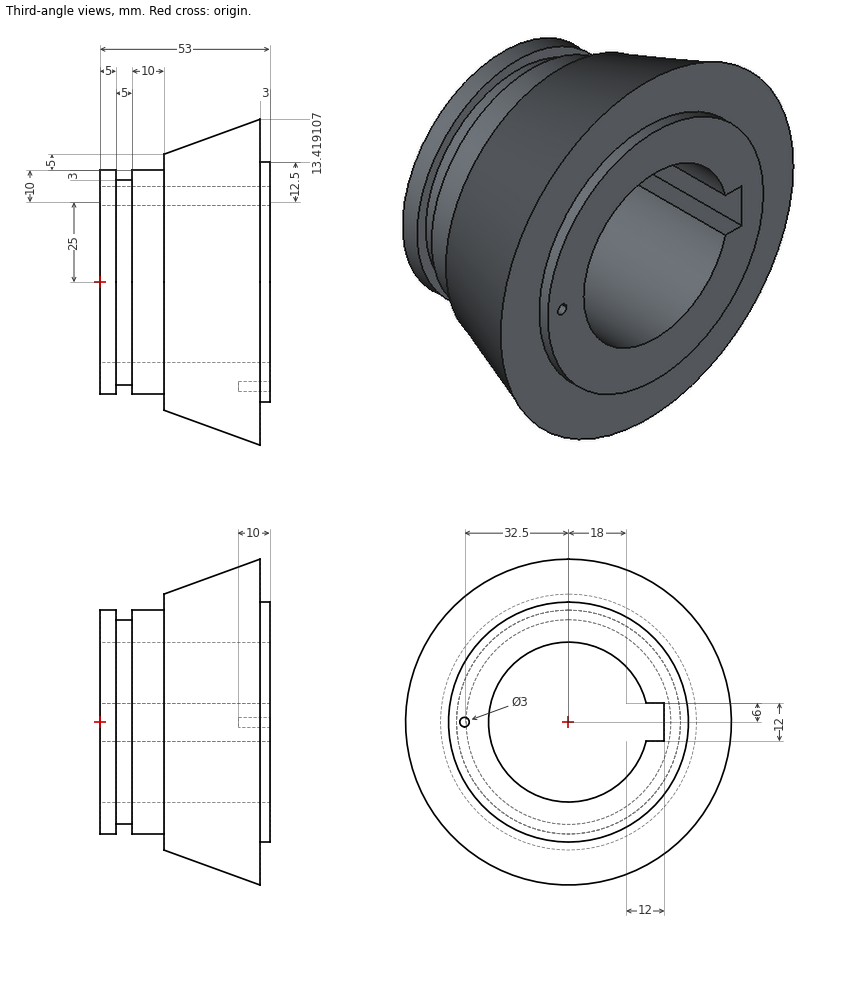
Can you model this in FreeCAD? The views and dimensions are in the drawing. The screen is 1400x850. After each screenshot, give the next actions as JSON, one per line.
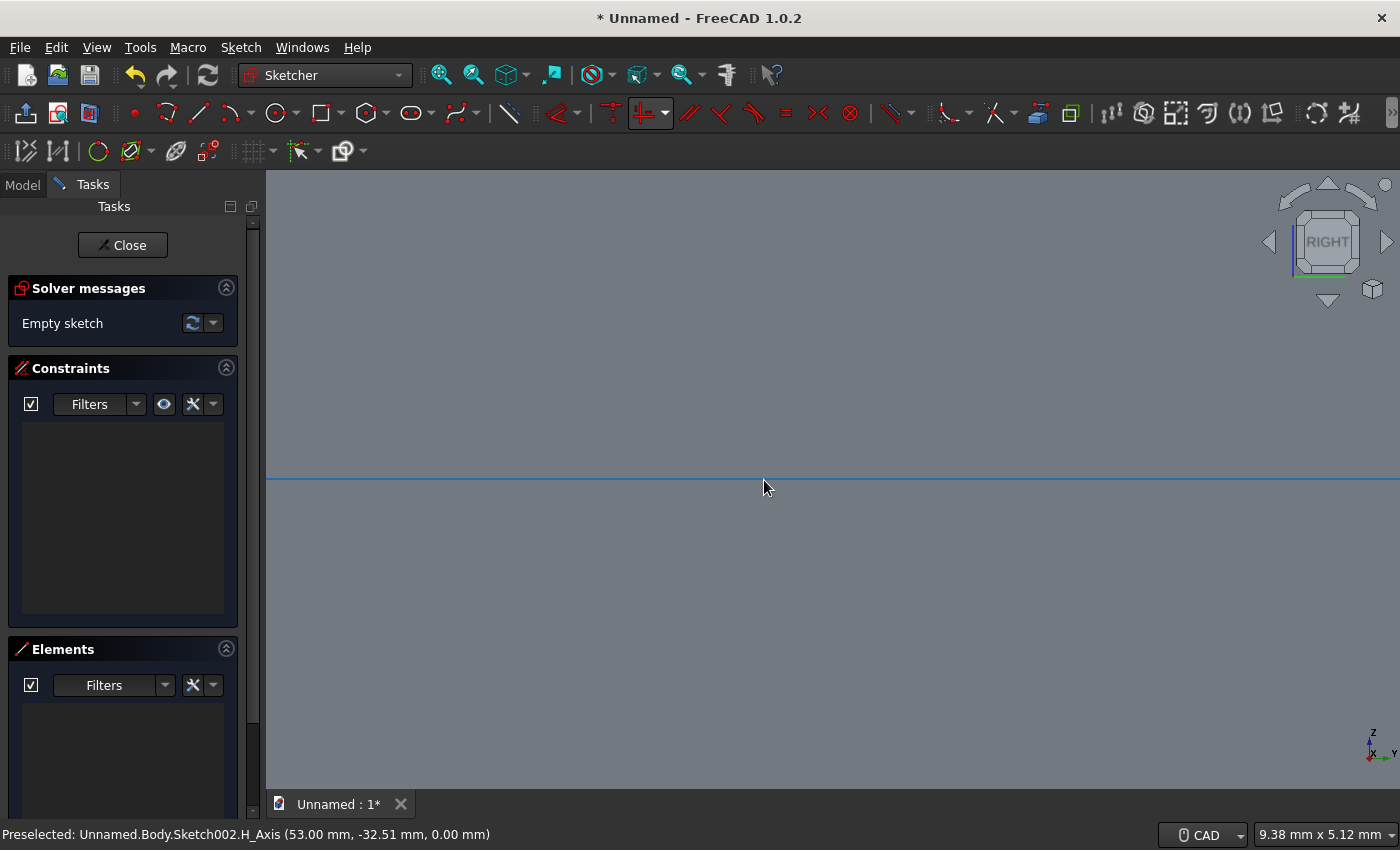
{"action": "left_click", "coordinate": [276, 114]}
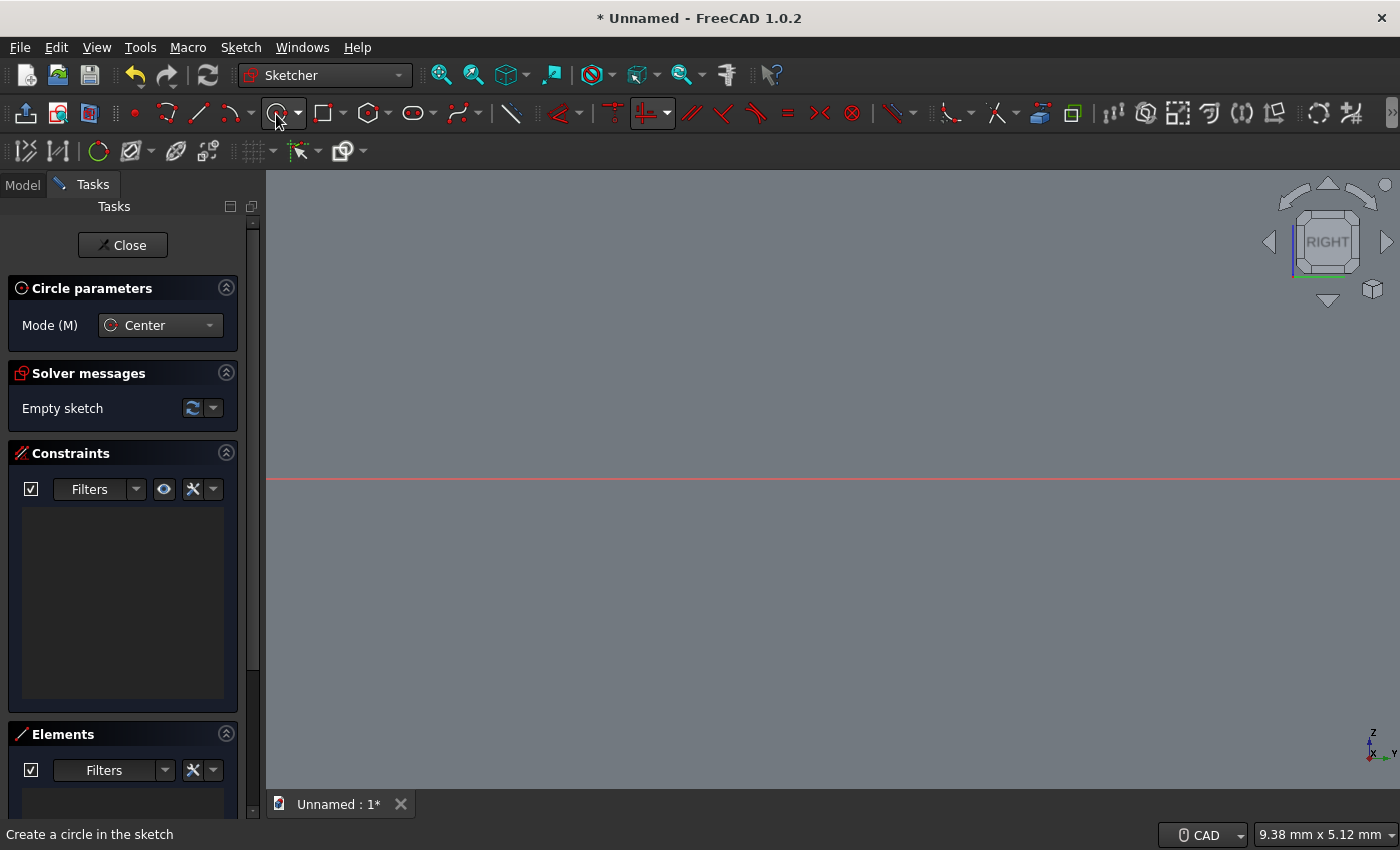
{"action": "left_click", "coordinate": [764, 479]}
{"action": "mouse_move", "coordinate": [893, 351]}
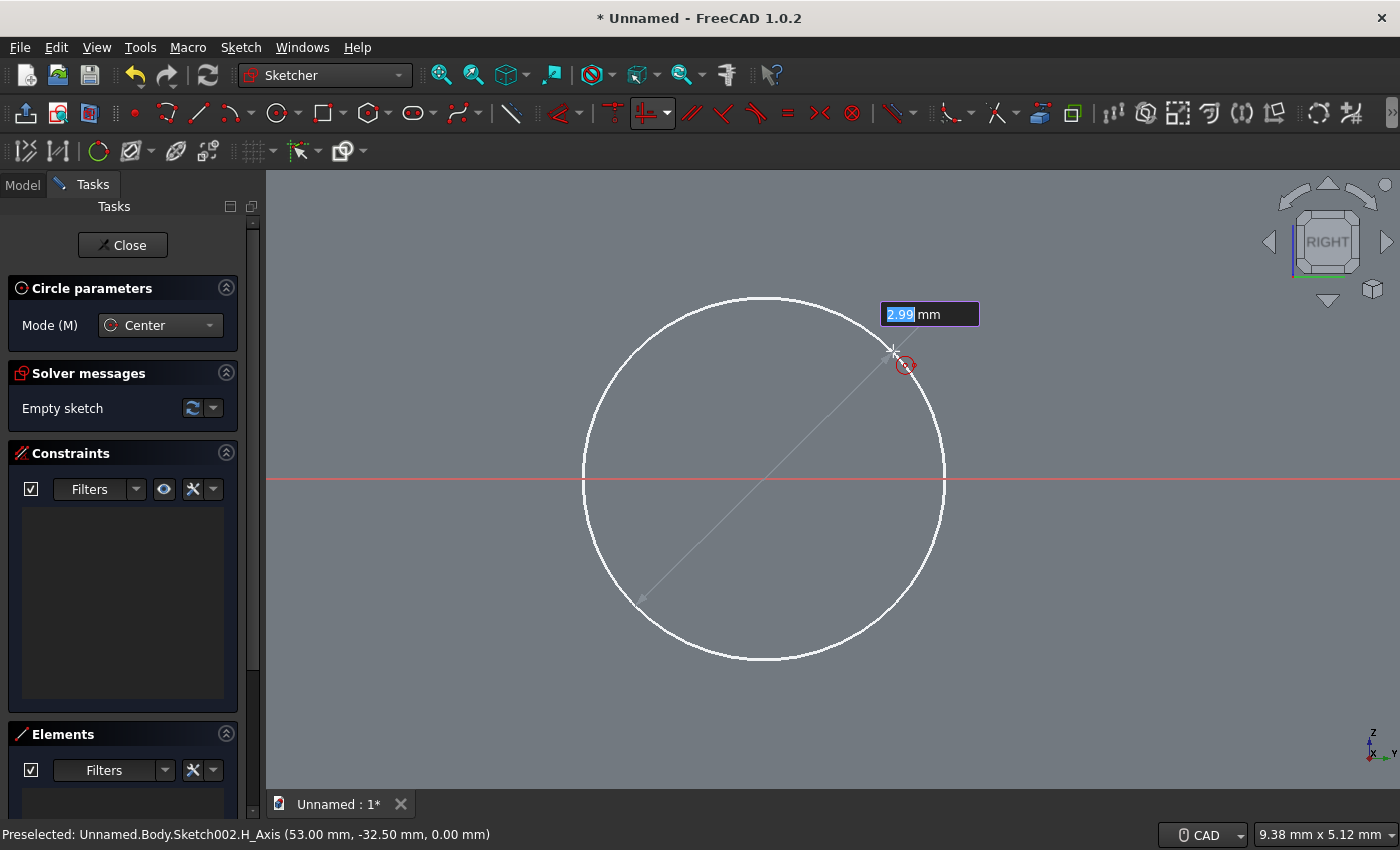
{"action": "type", "text": "3"}
{"action": "key", "text": "Return"}
{"action": "key", "text": "Escape"}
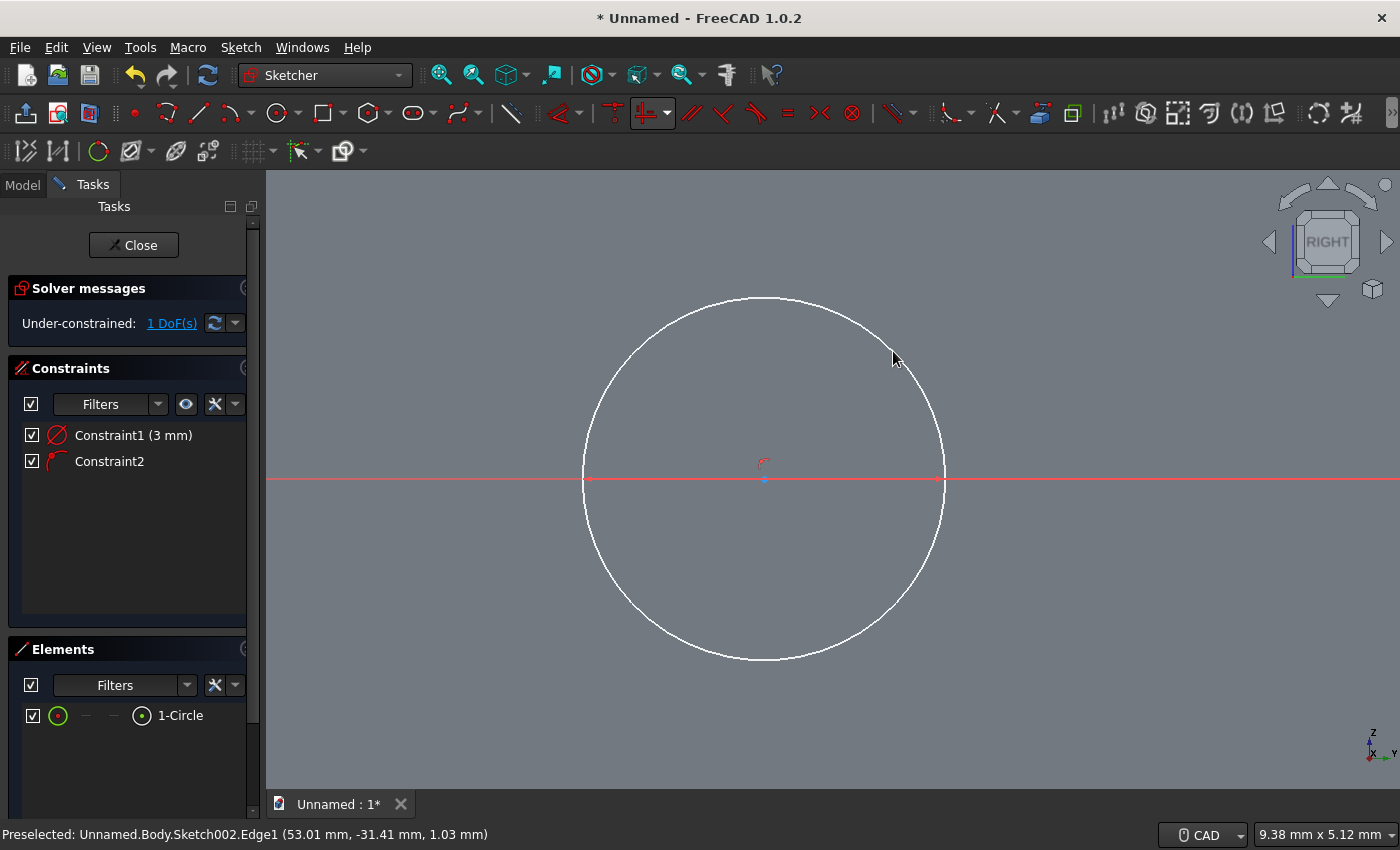
{"action": "left_click", "coordinate": [558, 114]}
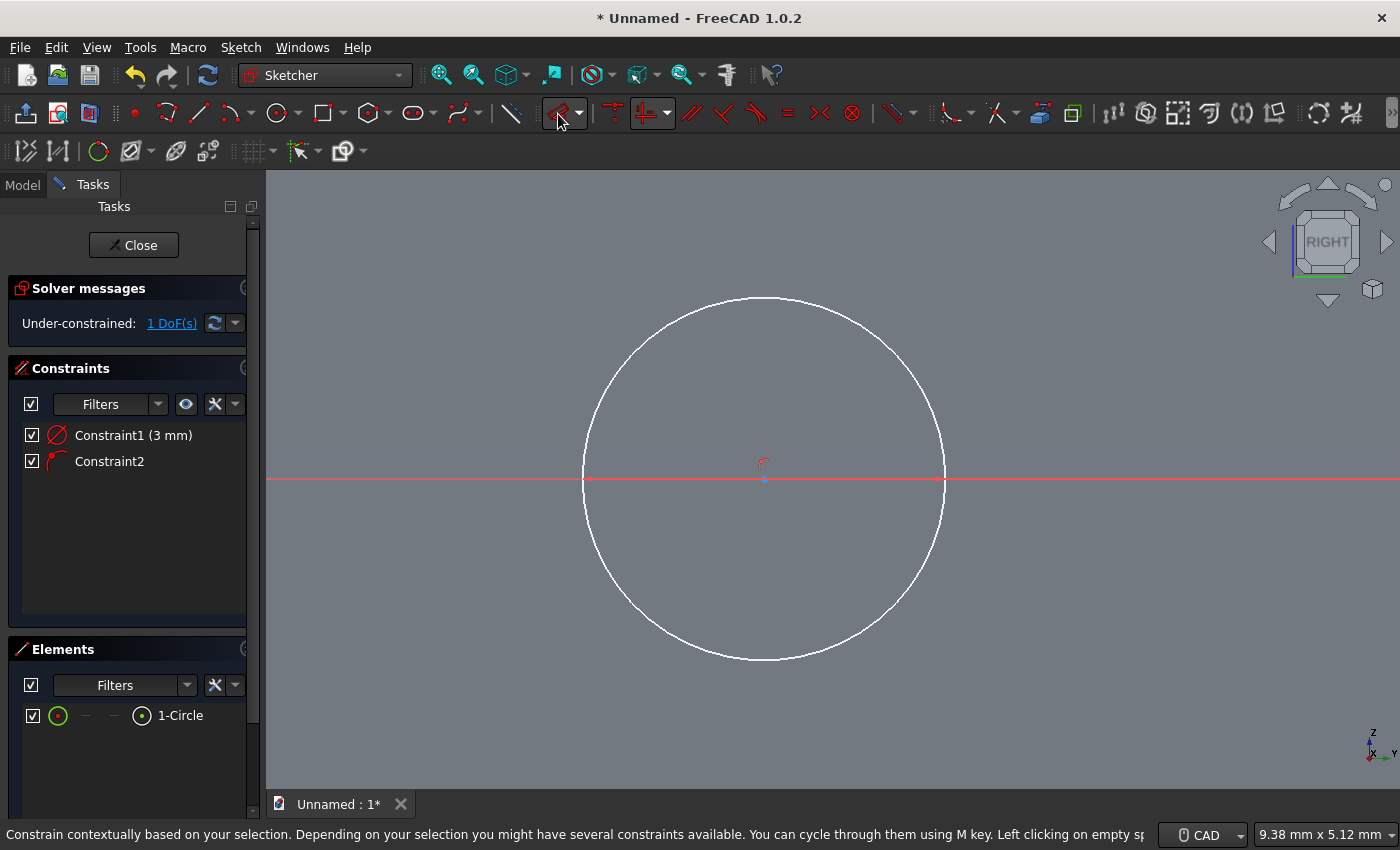
{"action": "left_click", "coordinate": [764, 479]}
{"action": "left_click", "coordinate": [1000, 513]}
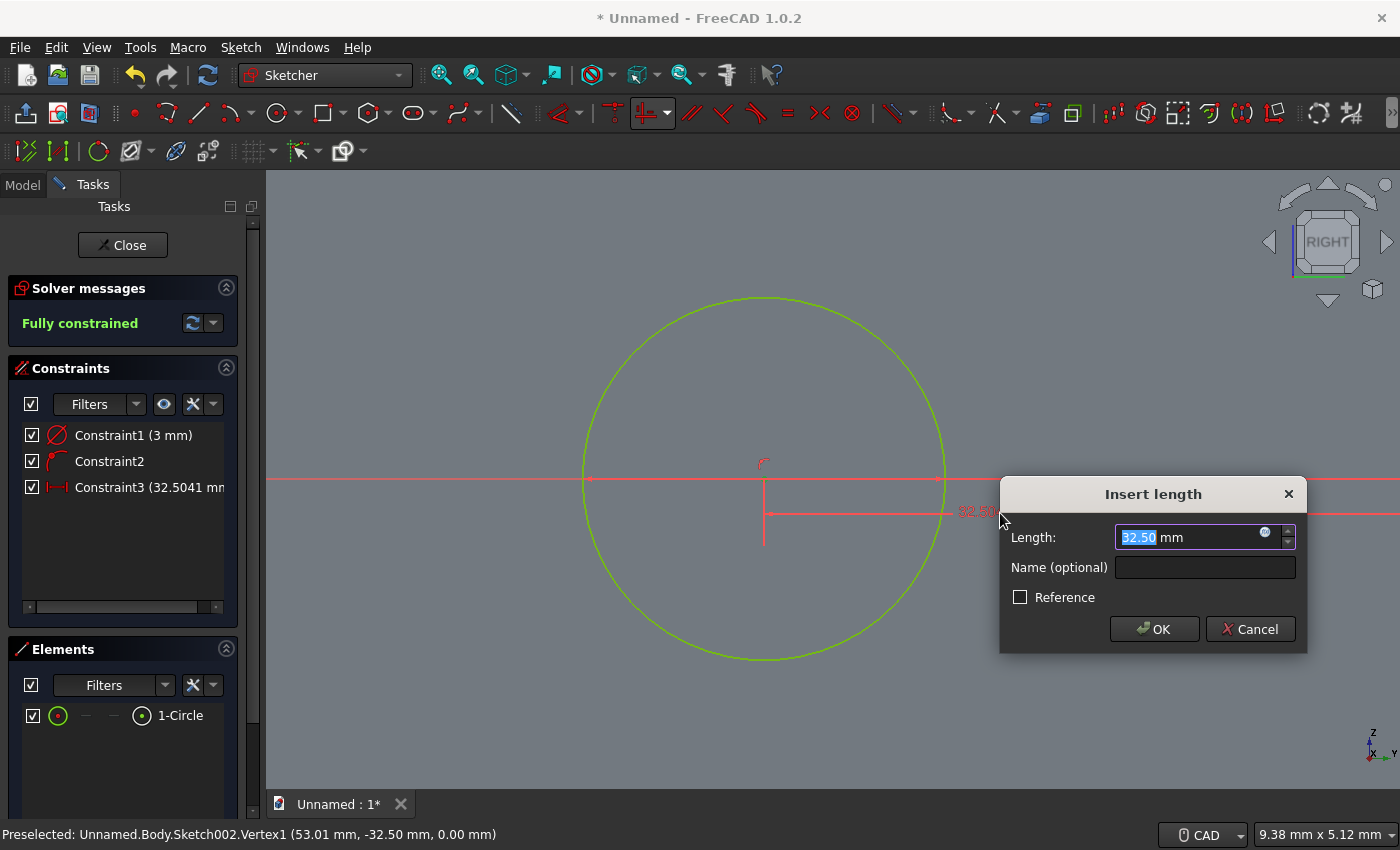
{"action": "type", "text": "32.5"}
{"action": "key", "text": "Return"}
{"action": "key", "text": "Escape"}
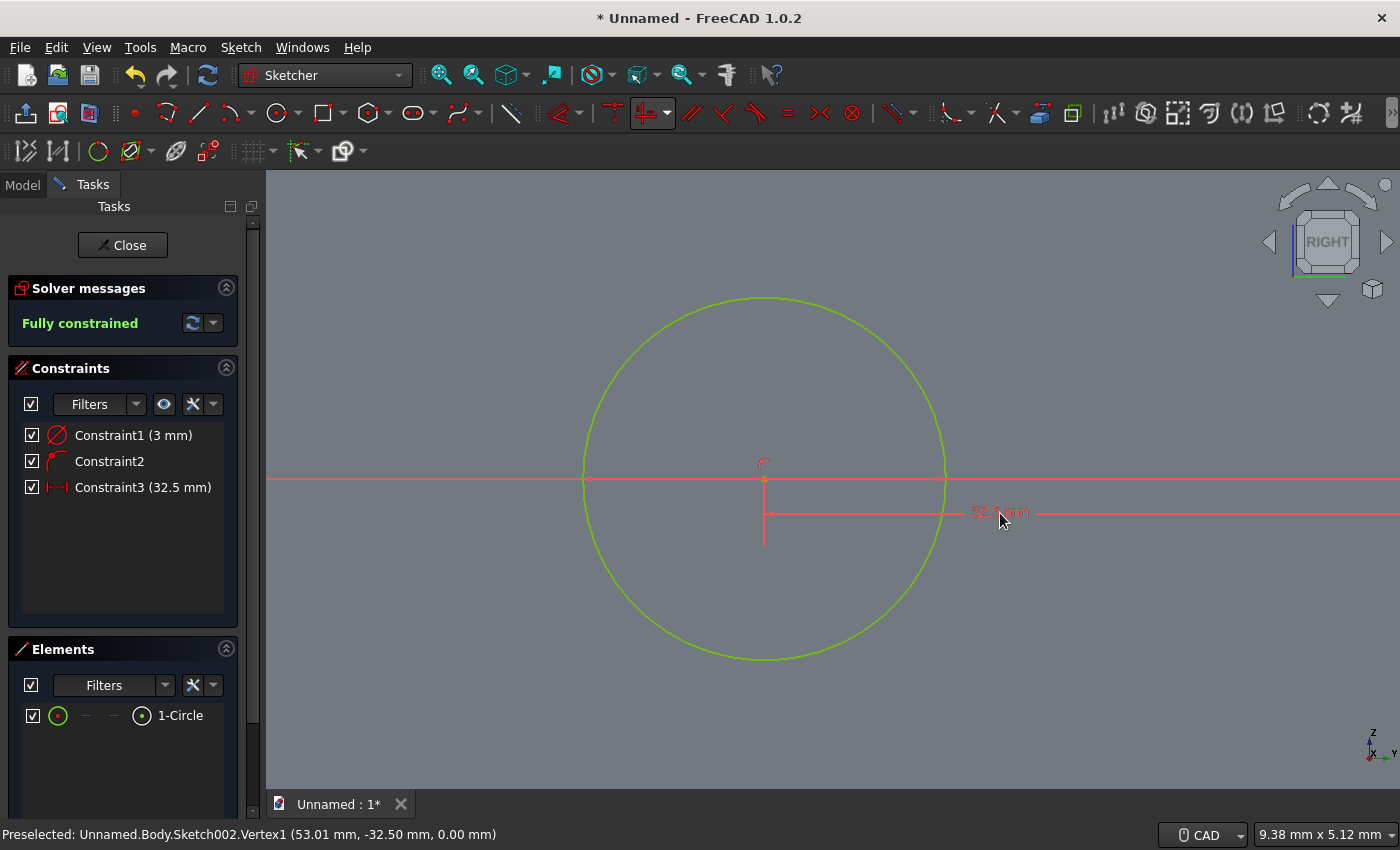
{"action": "left_click", "coordinate": [123, 245]}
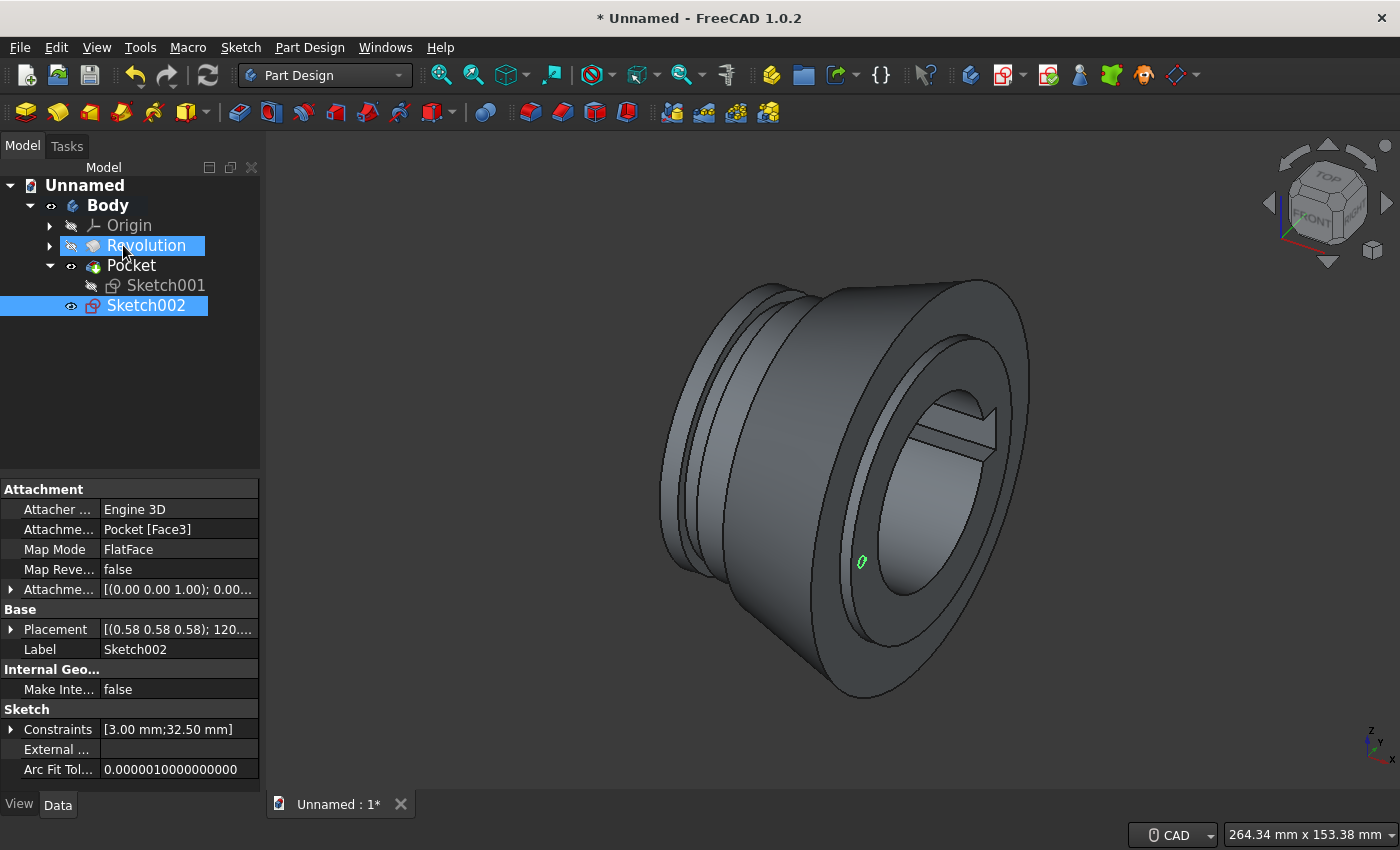
{"action": "left_click", "coordinate": [240, 112]}